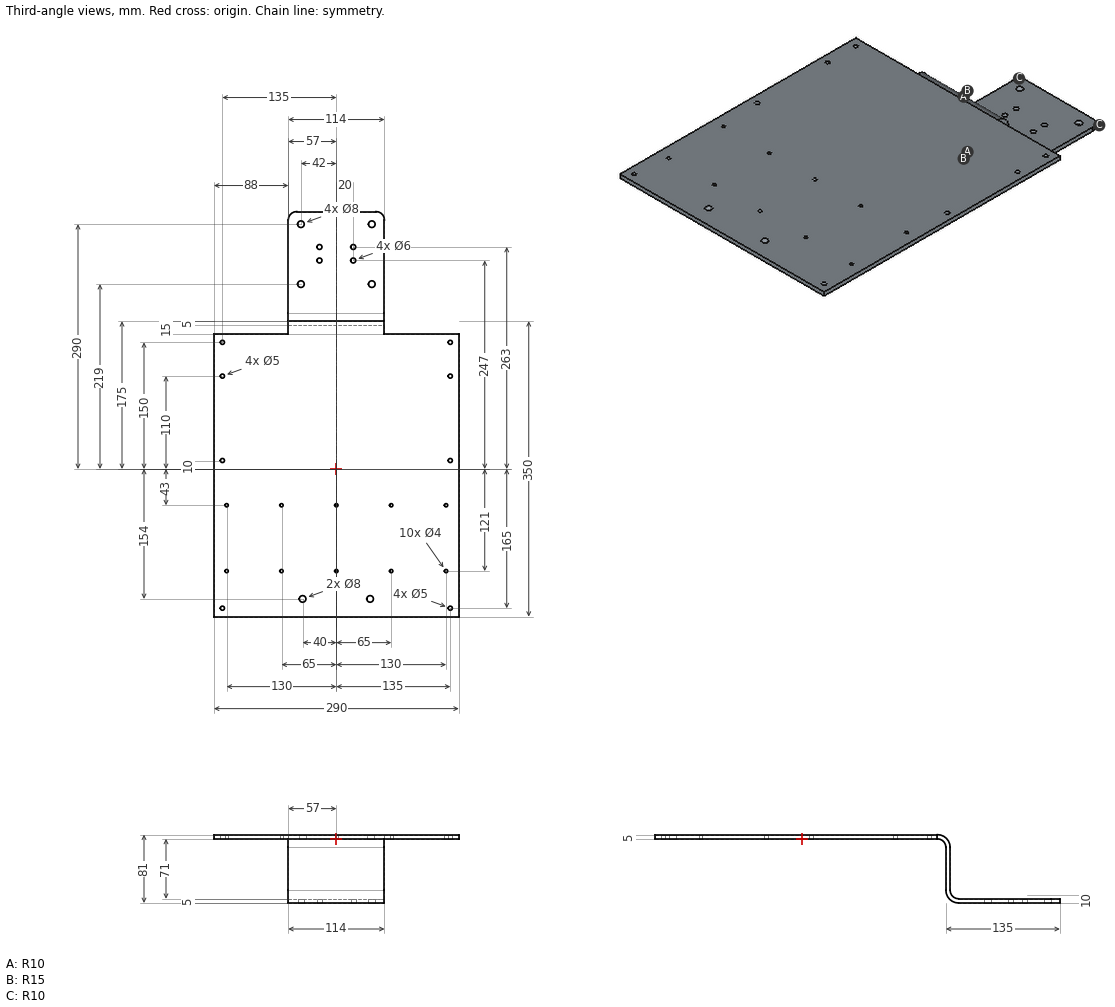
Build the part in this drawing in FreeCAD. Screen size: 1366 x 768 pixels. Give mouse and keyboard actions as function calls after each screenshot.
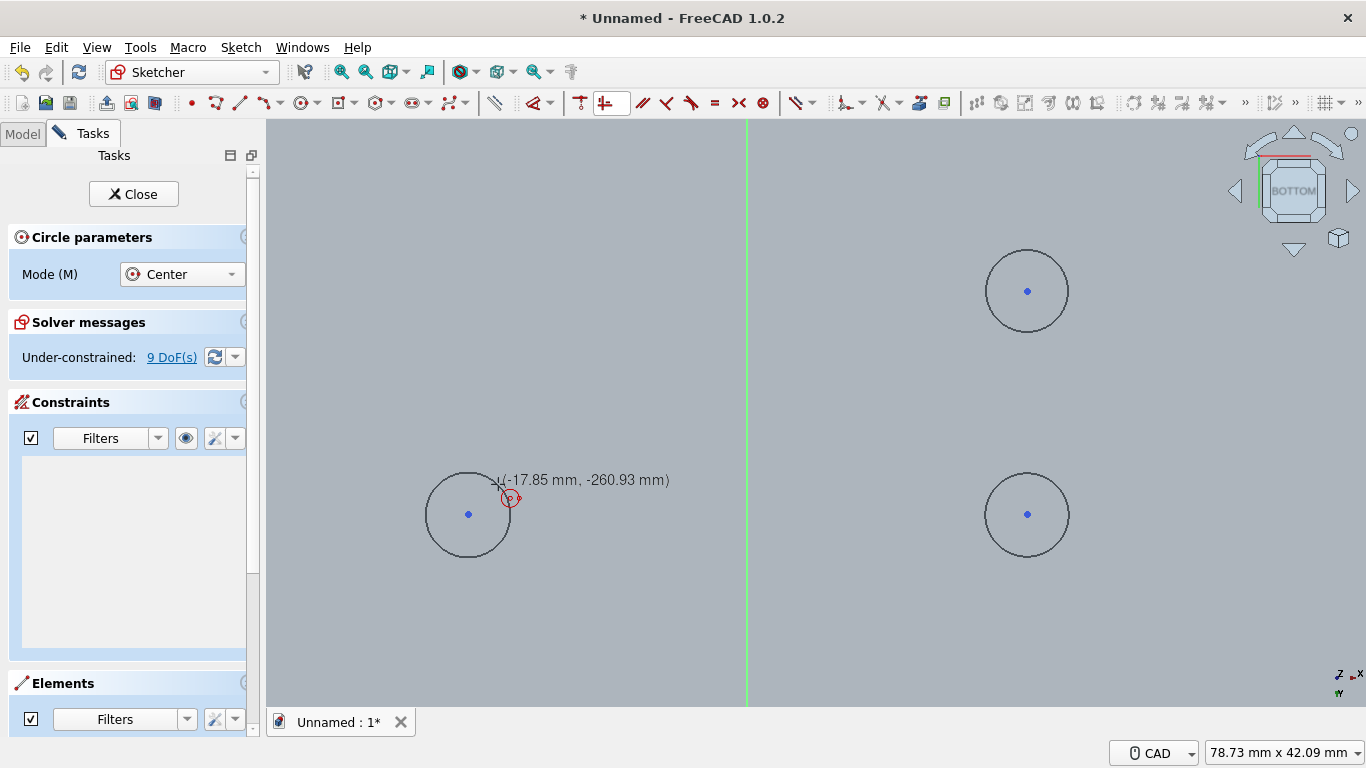
click(468, 290)
click(498, 261)
key(Escape)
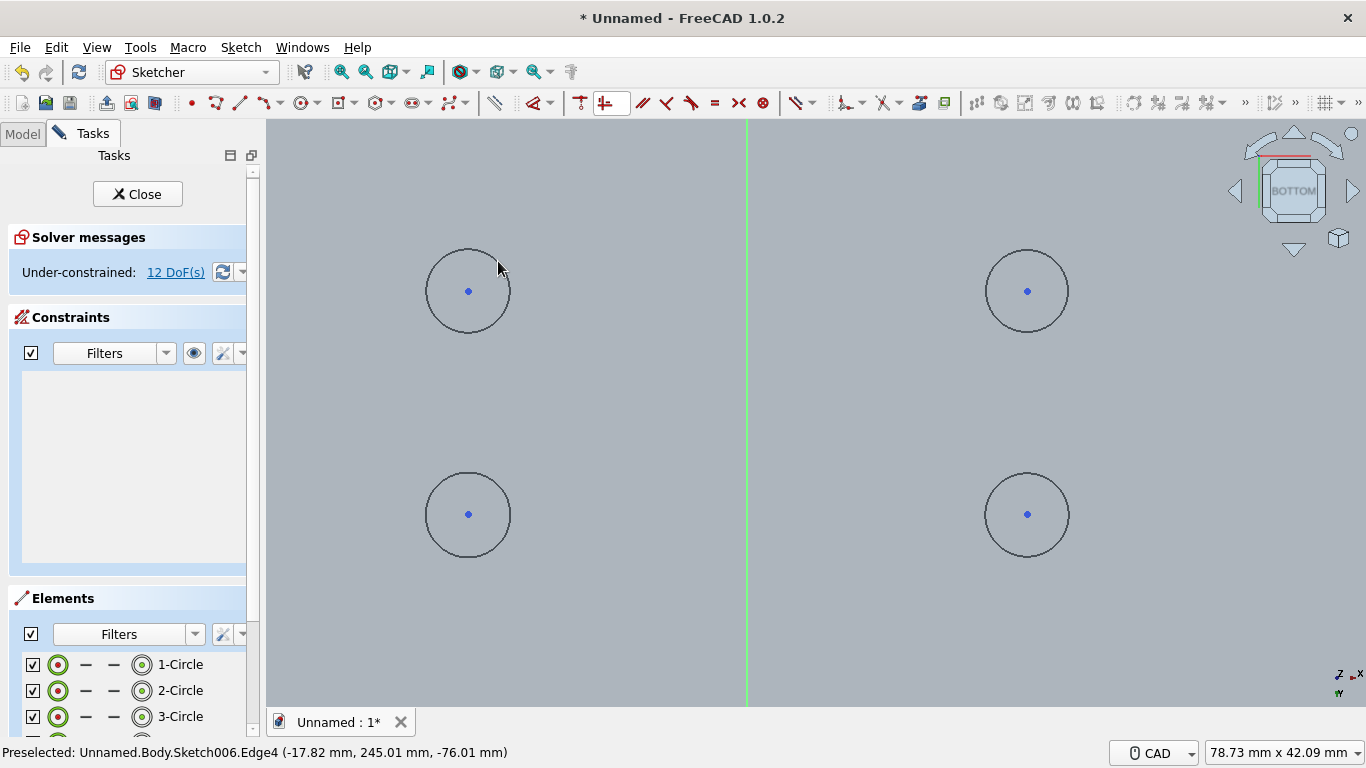
click(1056, 262)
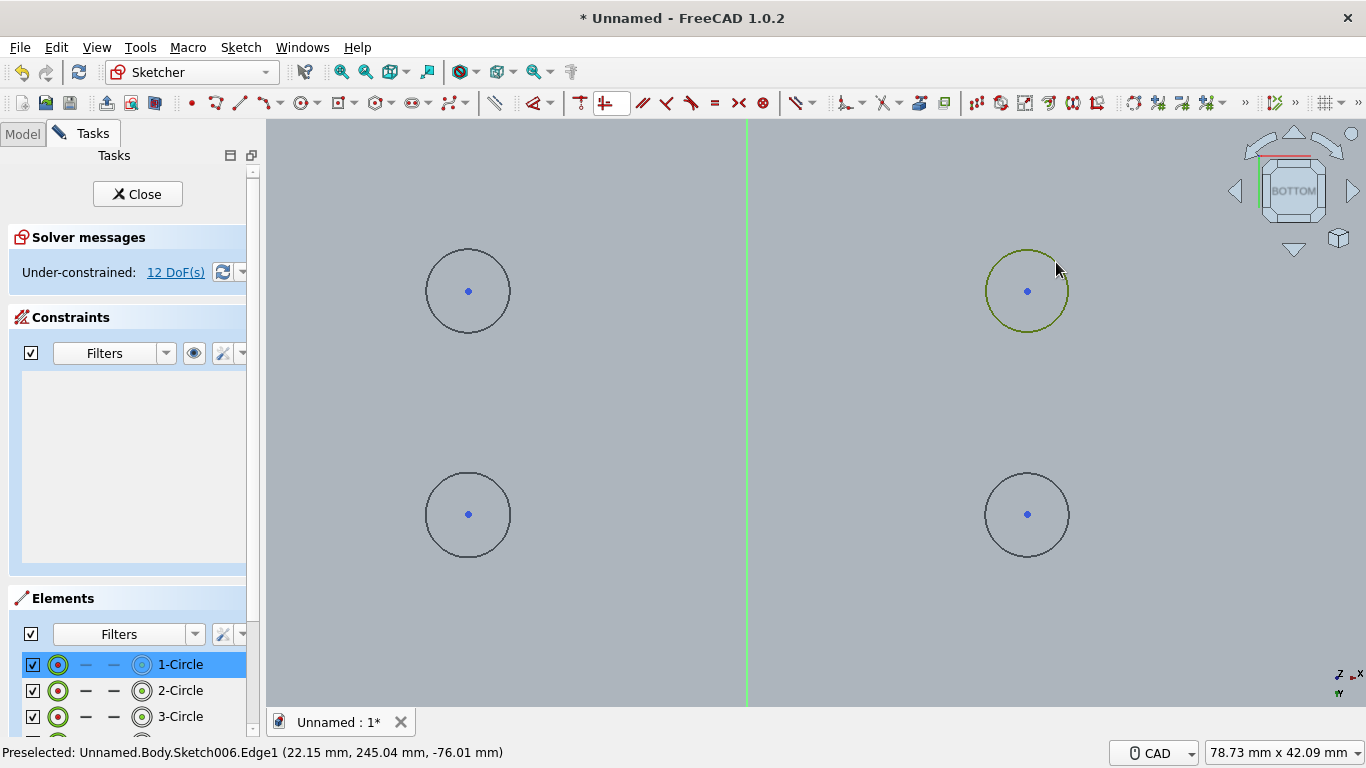
click(1056, 485)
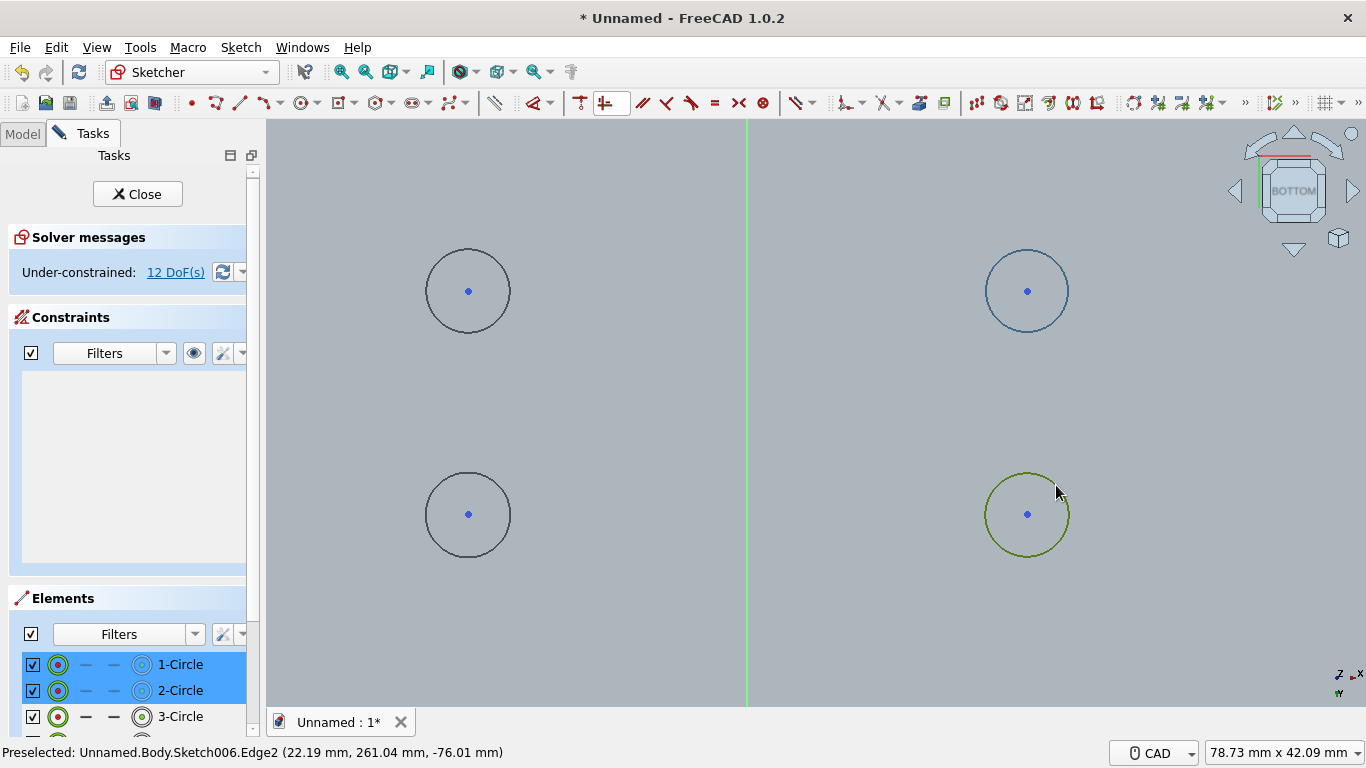
click(498, 485)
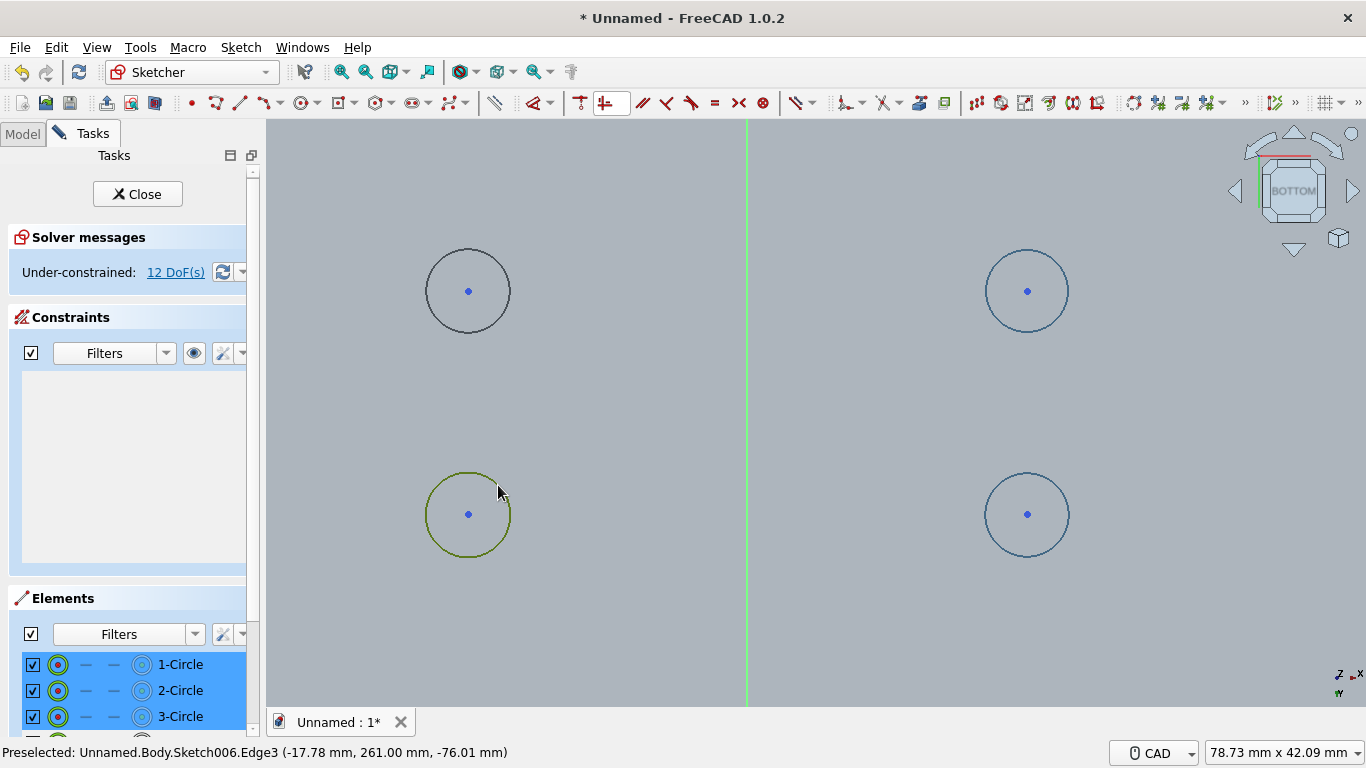
click(497, 261)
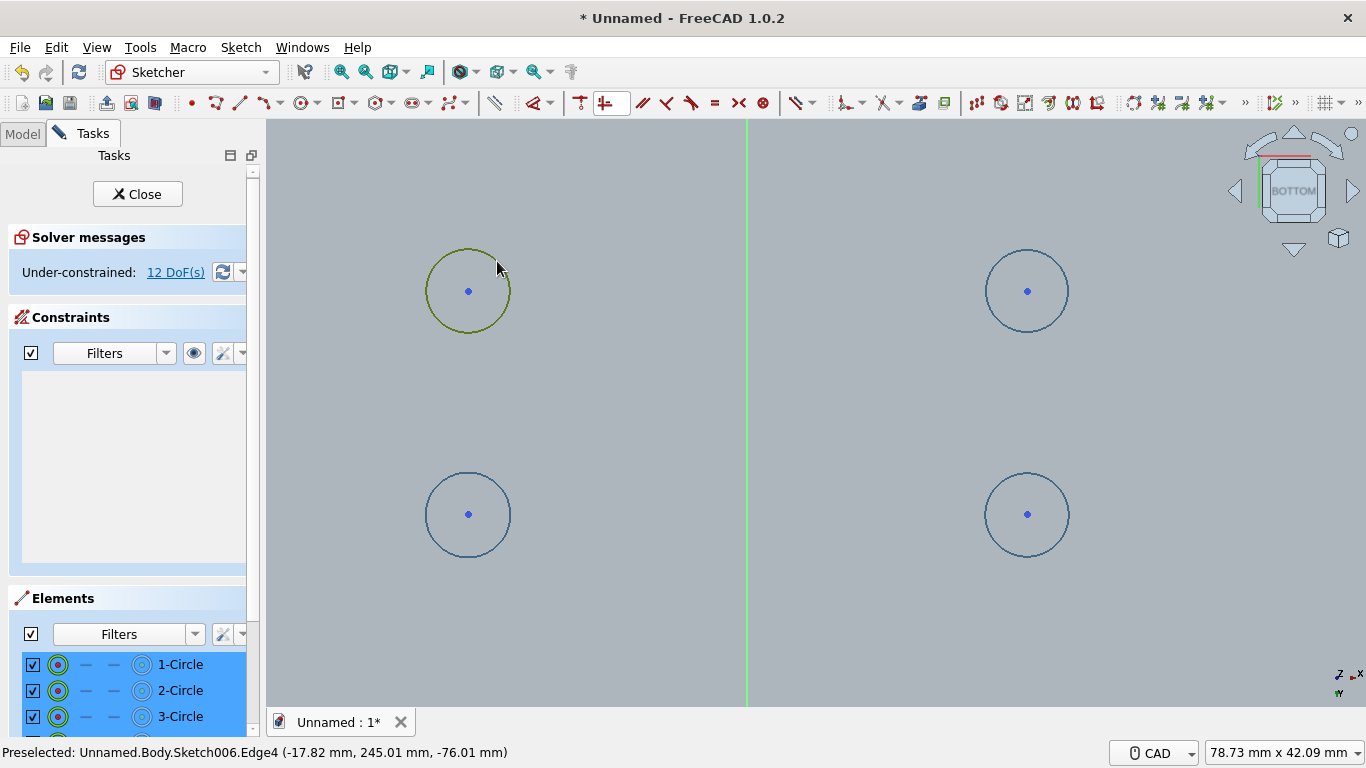
click(716, 104)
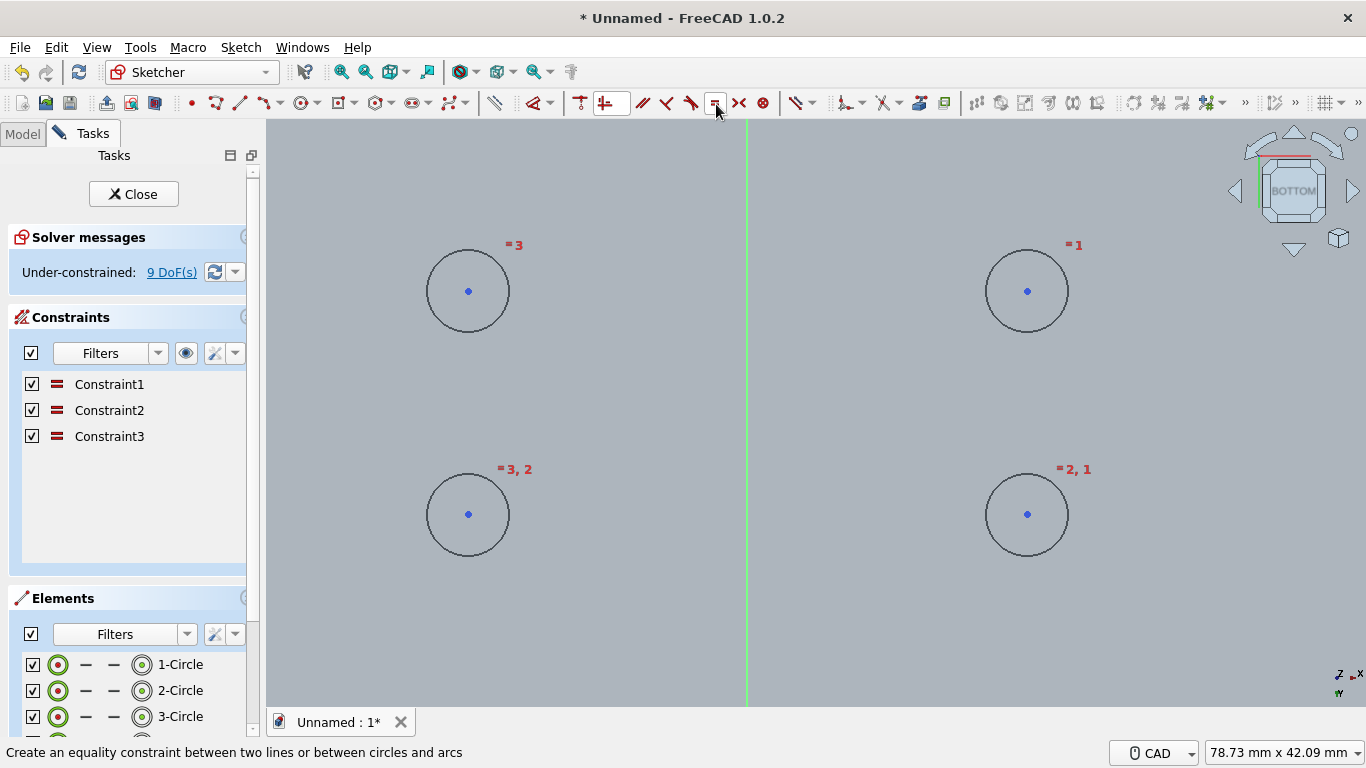
click(1027, 515)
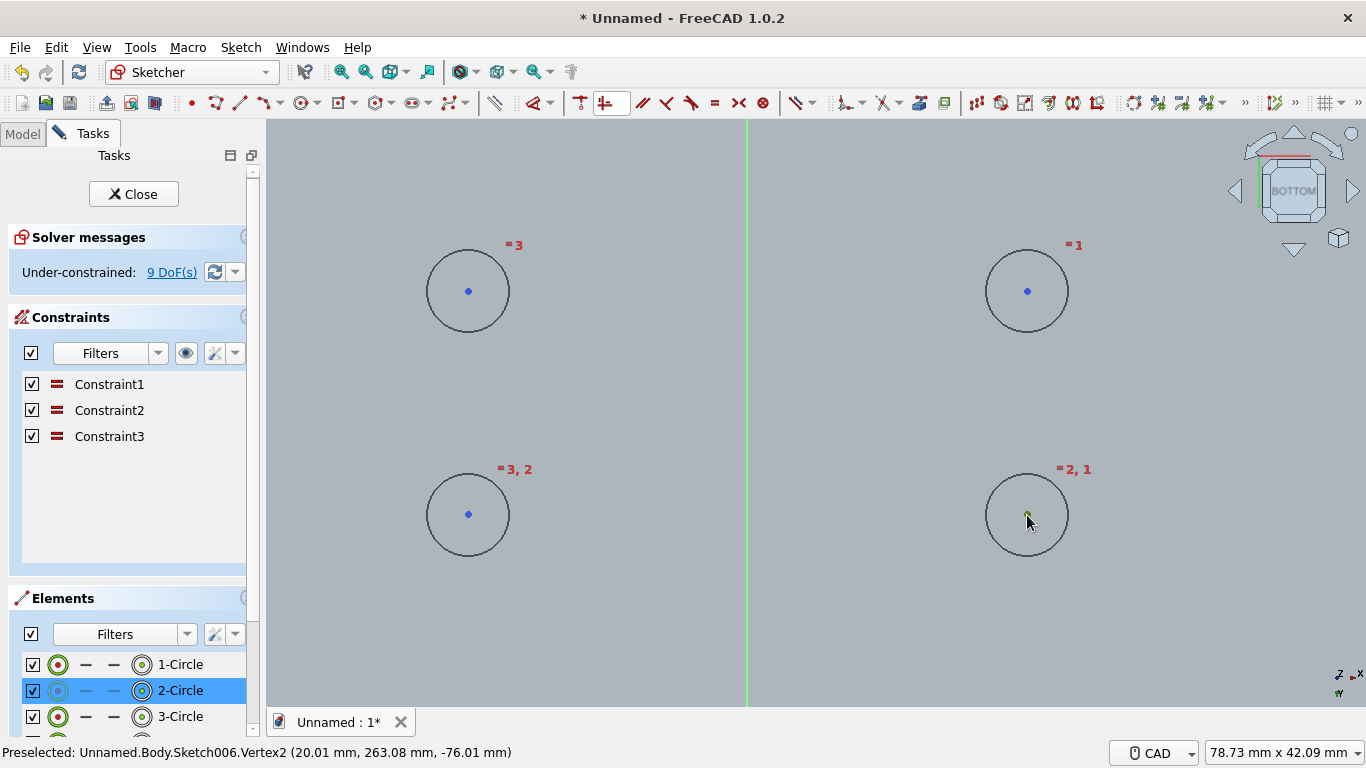
click(468, 515)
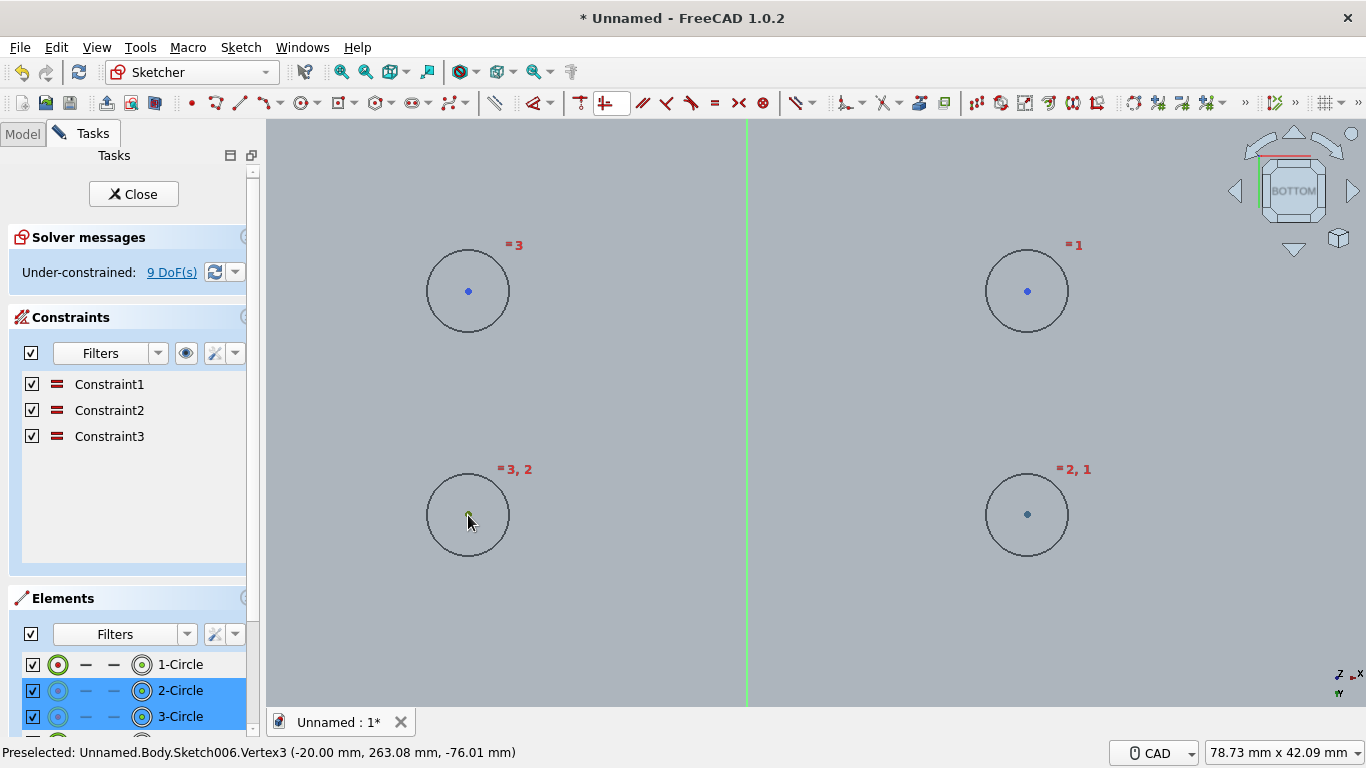
click(747, 641)